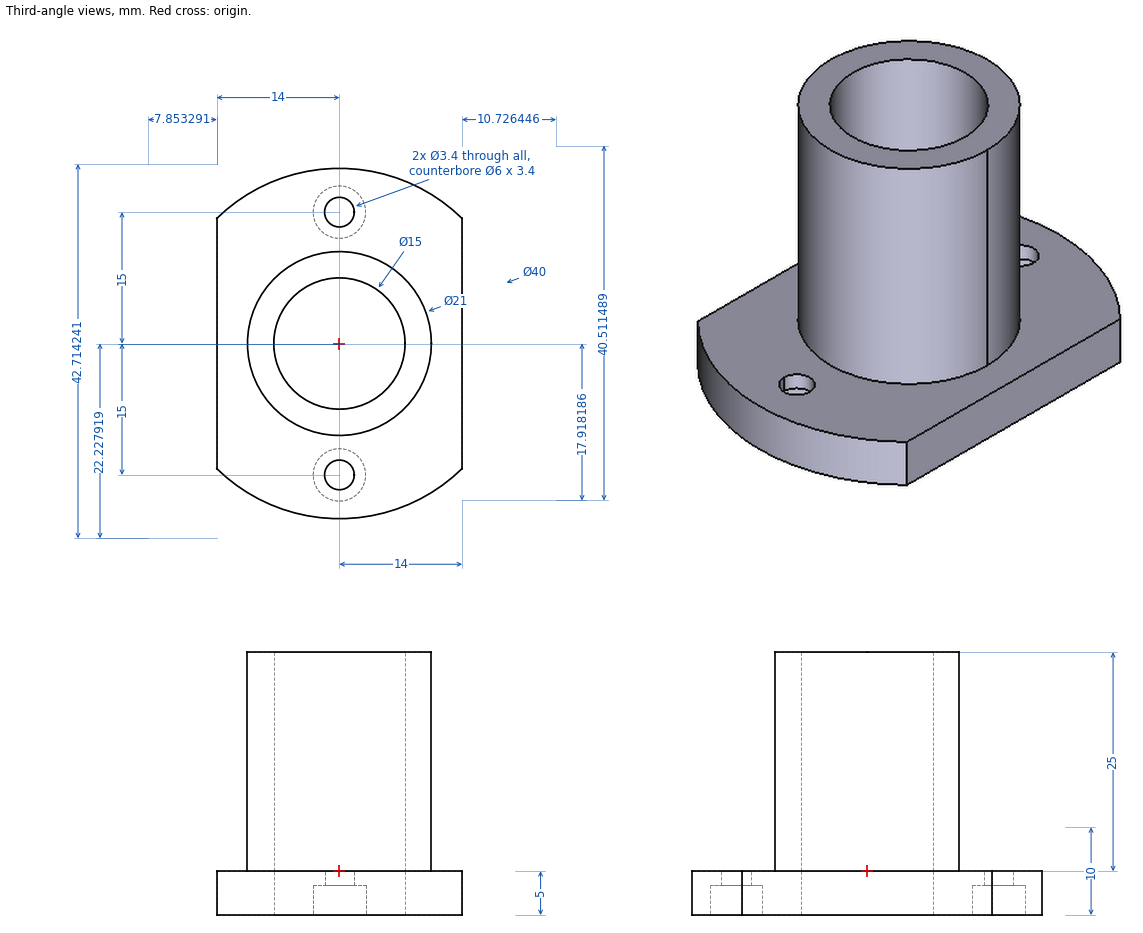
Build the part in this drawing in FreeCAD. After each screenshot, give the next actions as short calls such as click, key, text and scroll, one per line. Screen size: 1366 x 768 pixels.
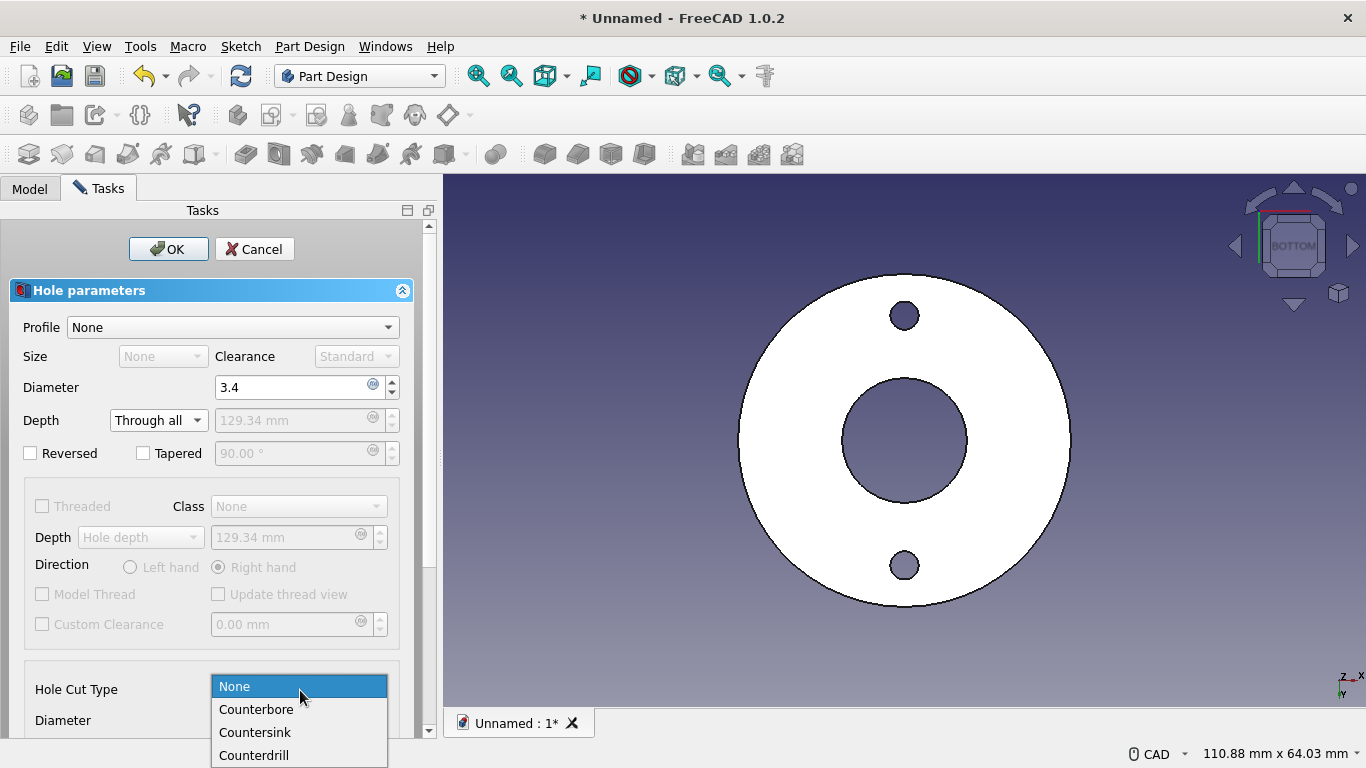
click(298, 710)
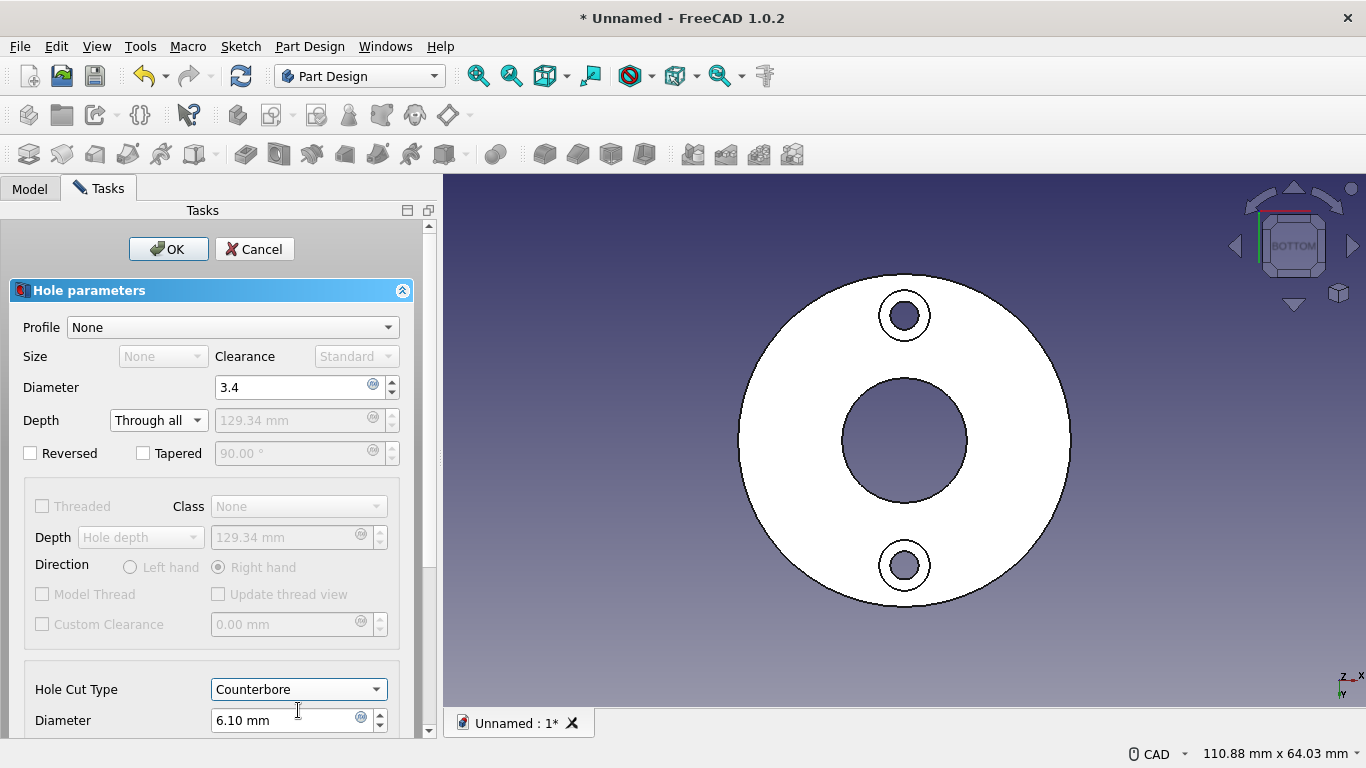
triple_click(292, 720)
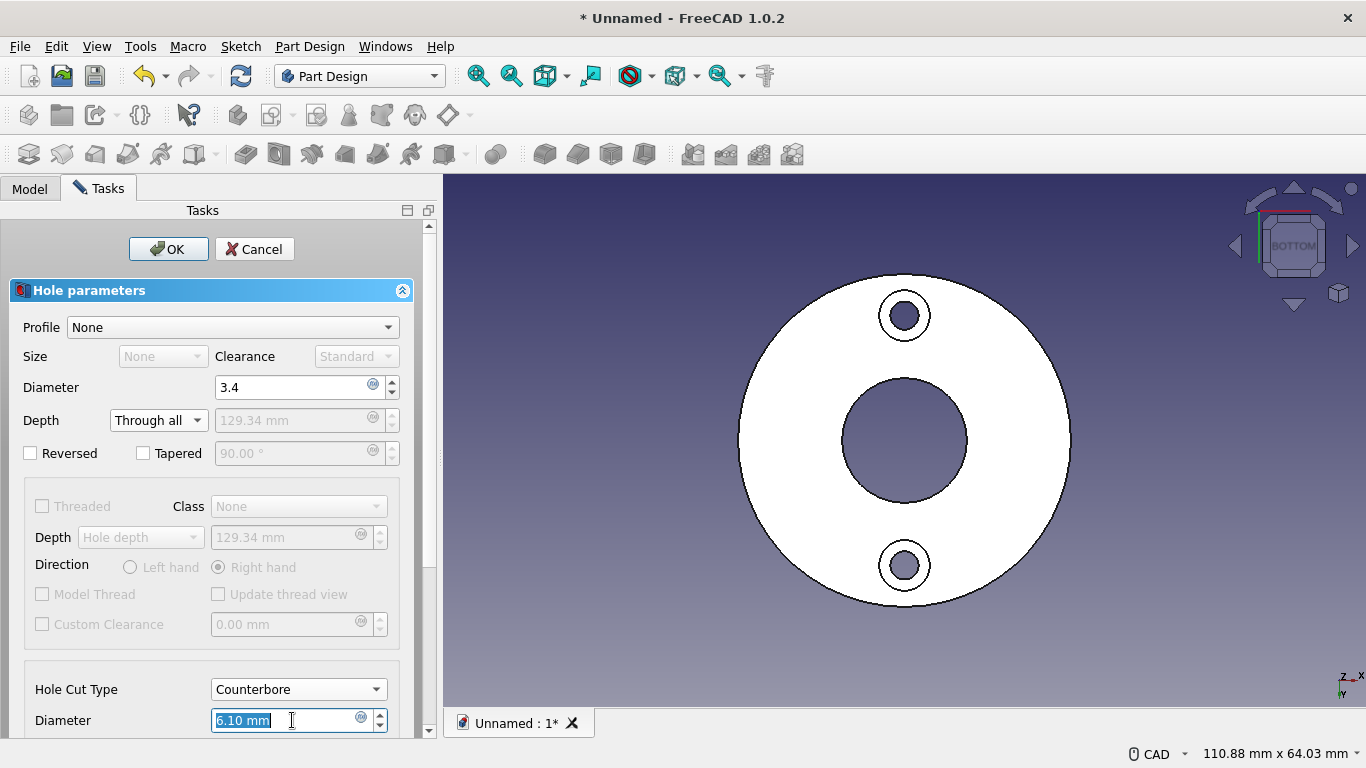
text(6)
key(Tab)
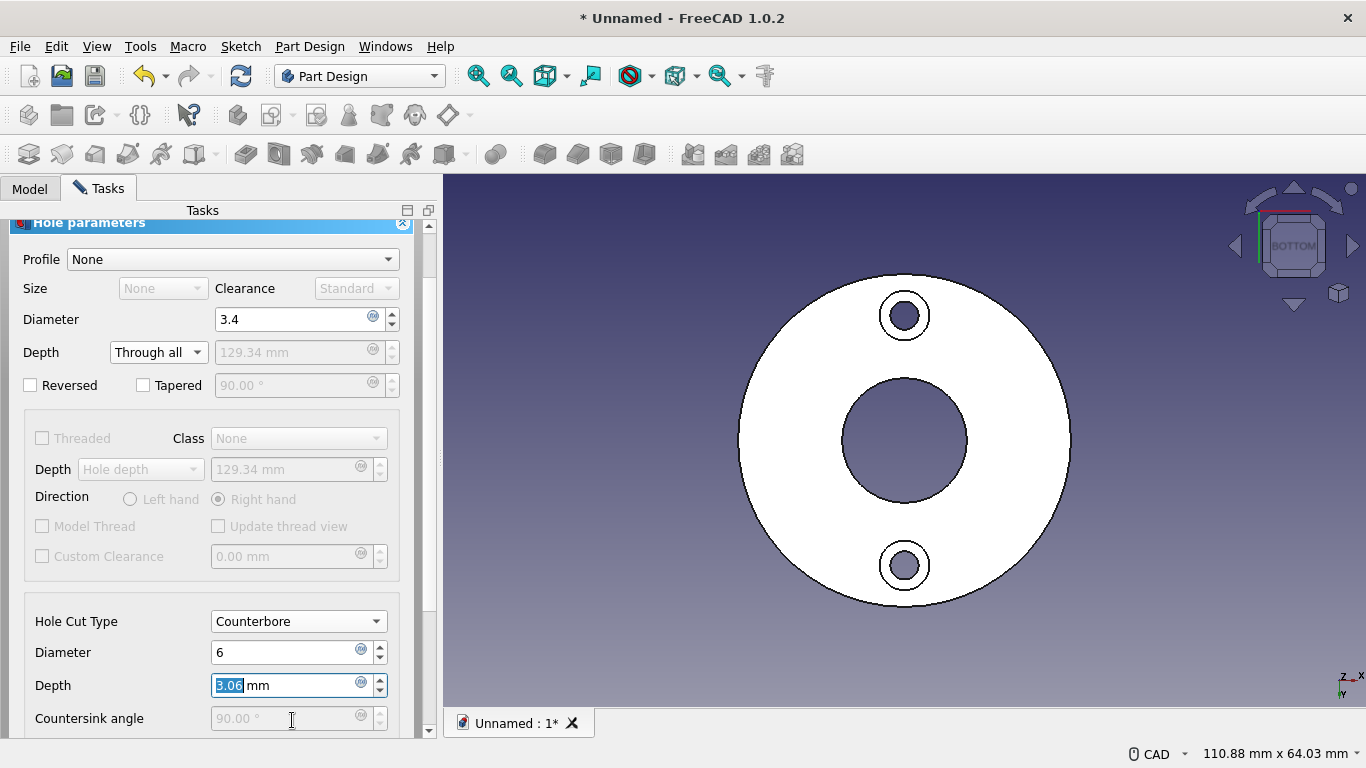
text(3.4)
key(Tab)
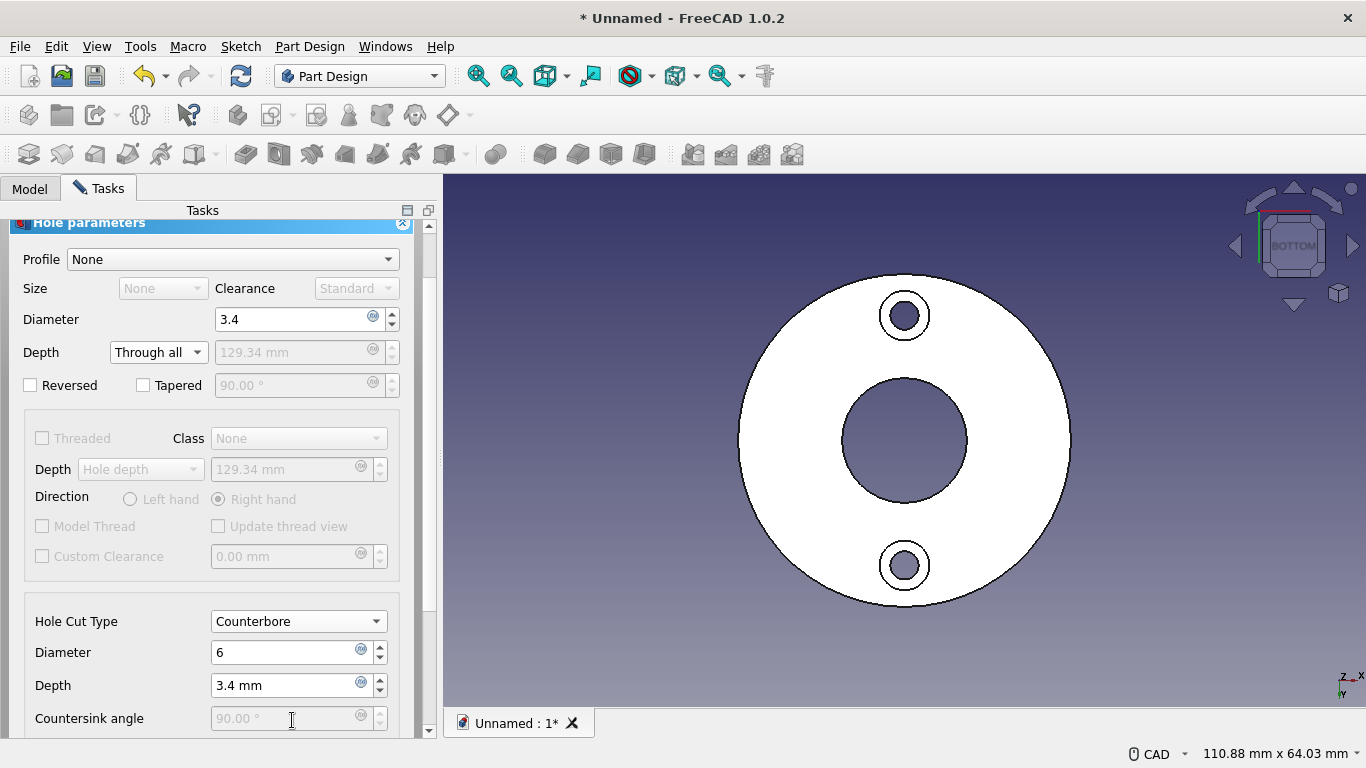
scroll(429, 479, up, 2)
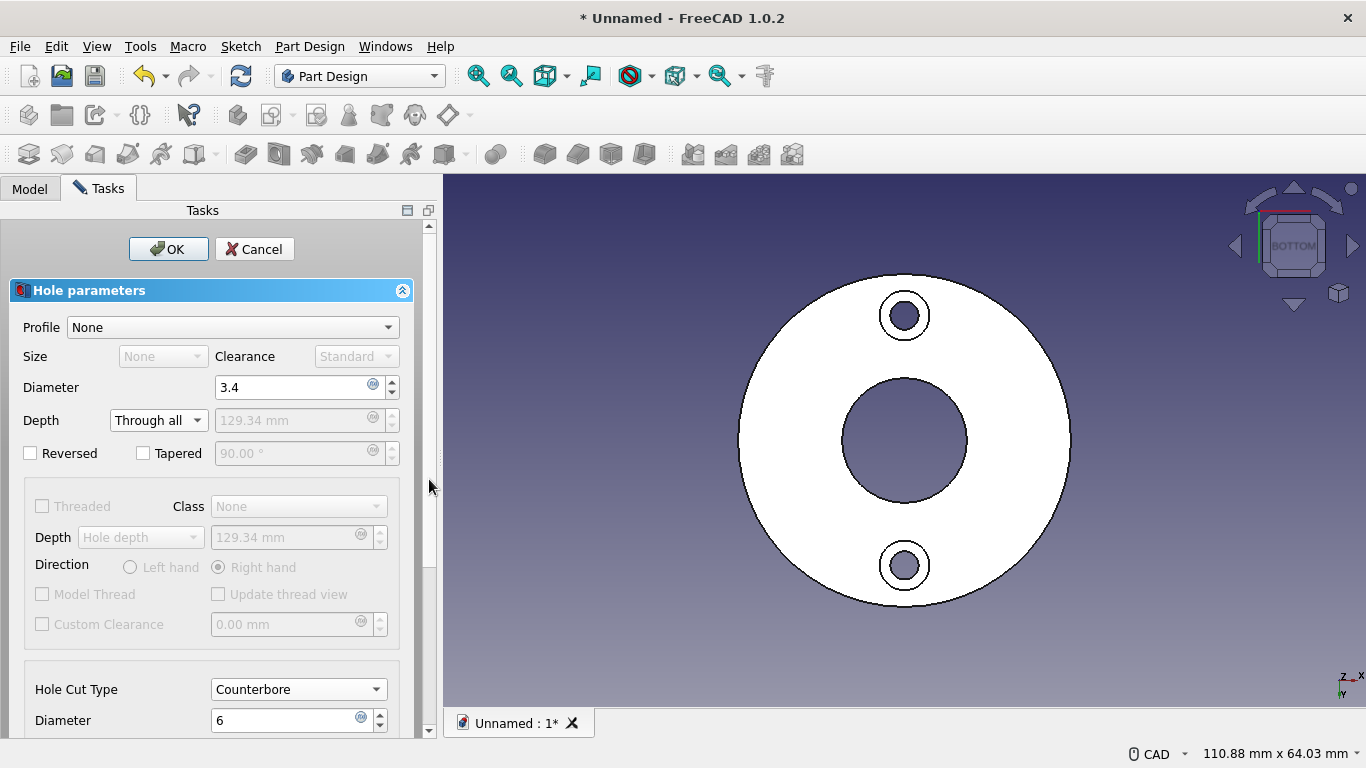
click(169, 249)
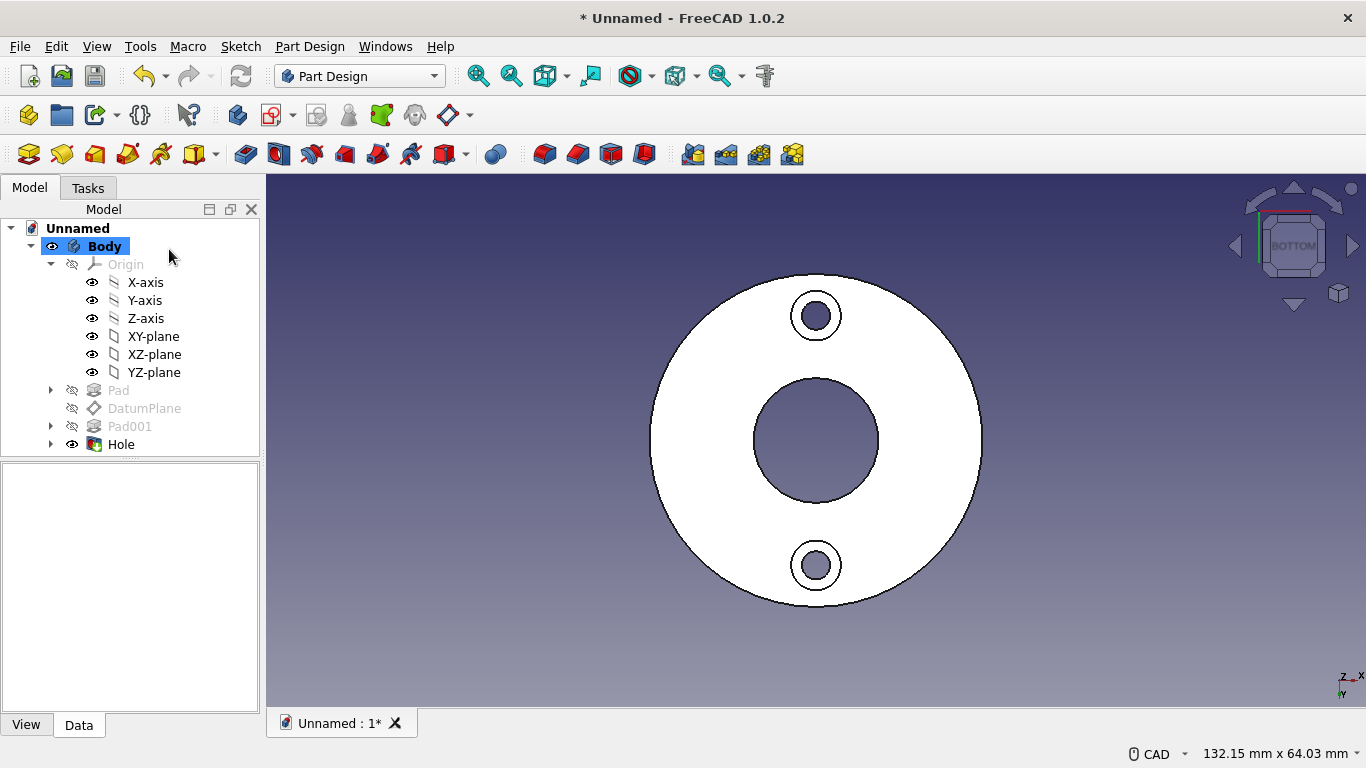
click(721, 487)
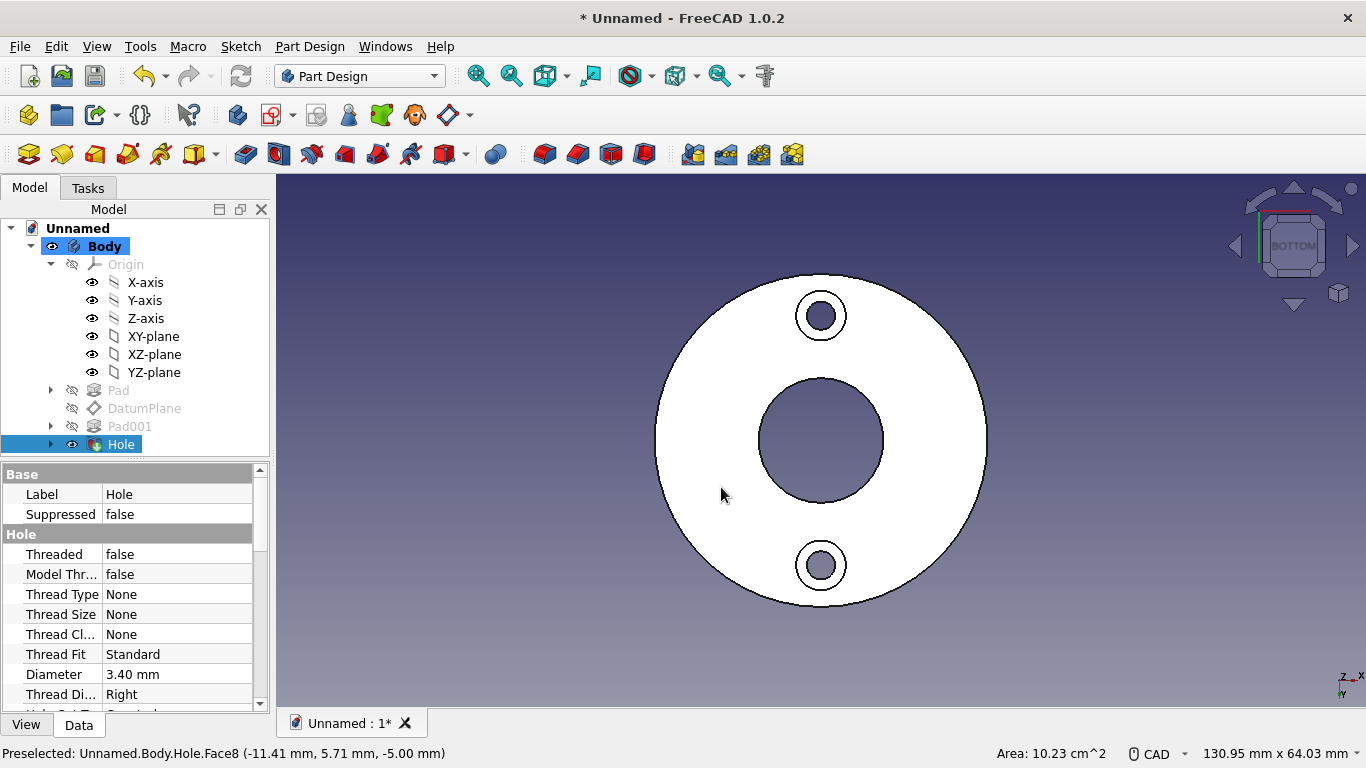
click(270, 116)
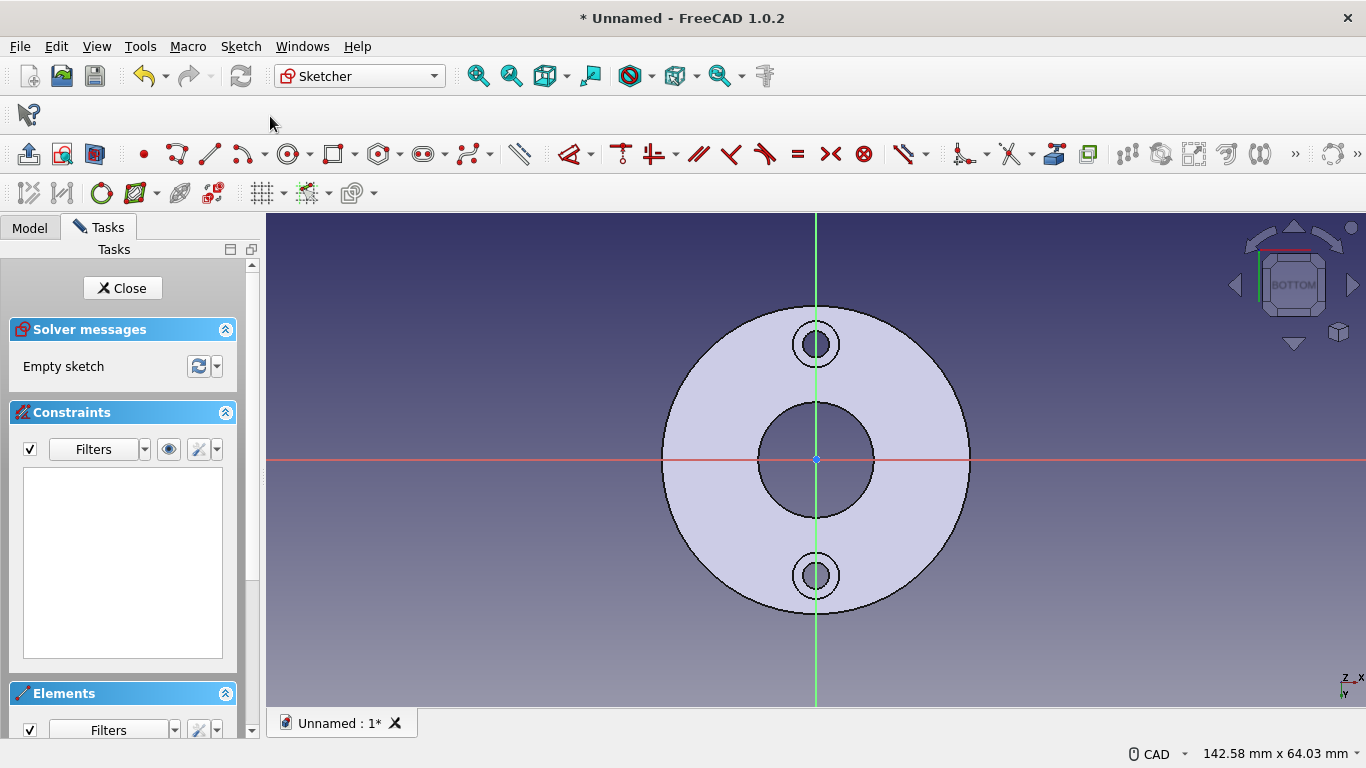
click(332, 154)